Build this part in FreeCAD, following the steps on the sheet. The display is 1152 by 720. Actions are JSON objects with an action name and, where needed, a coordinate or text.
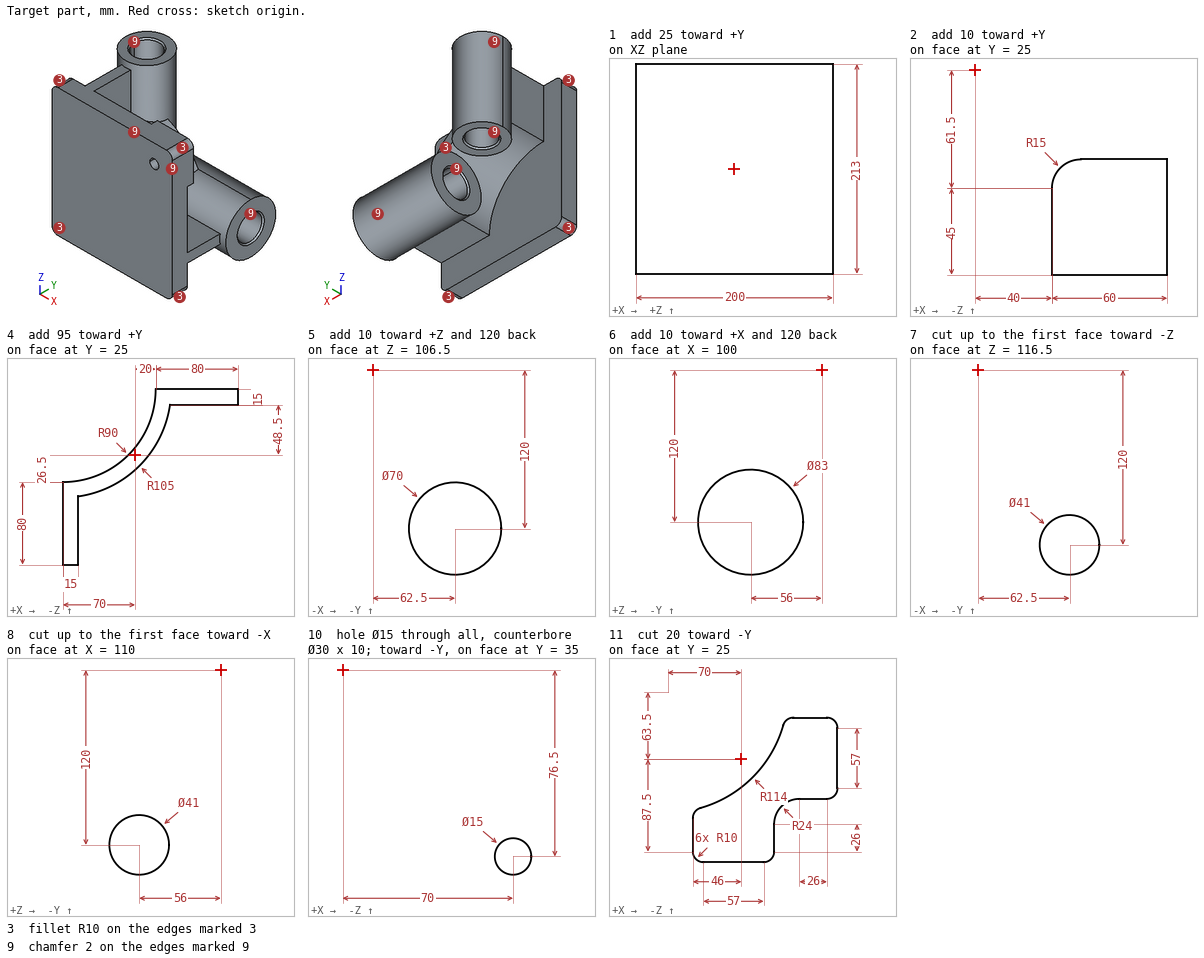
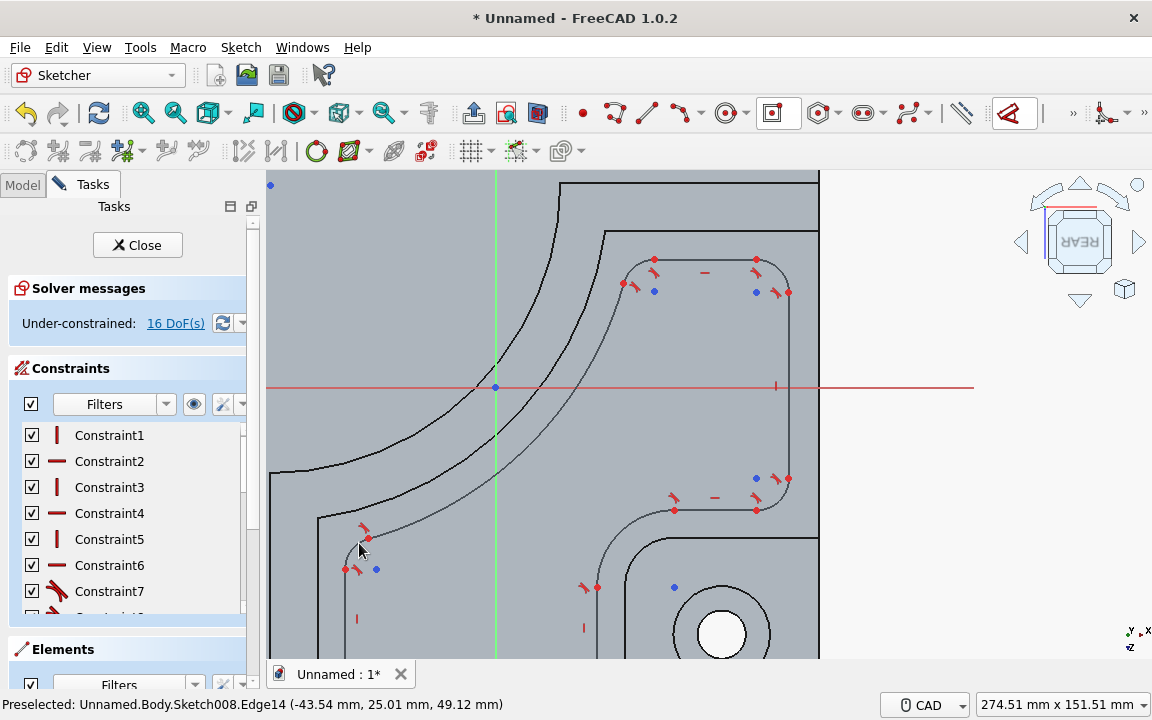
{"action": "scroll", "coordinate": [787, 279], "scroll_direction": "down", "scroll_amount": 2}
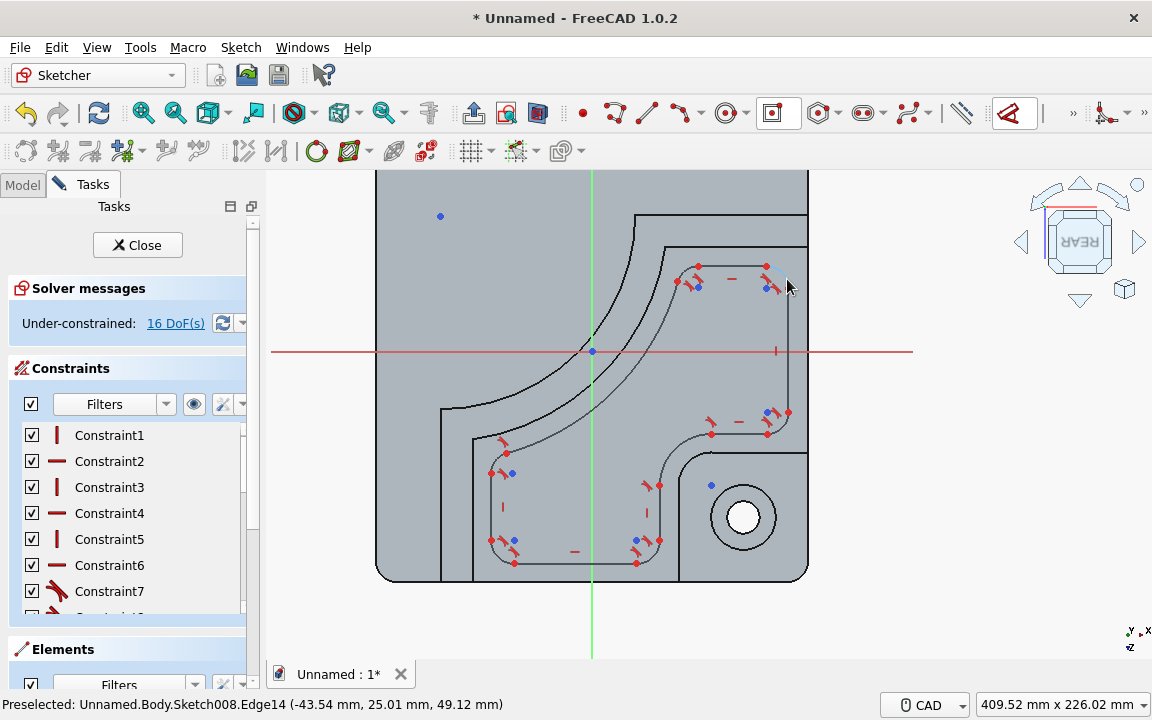
{"action": "scroll", "coordinate": [494, 551], "scroll_direction": "up", "scroll_amount": 2}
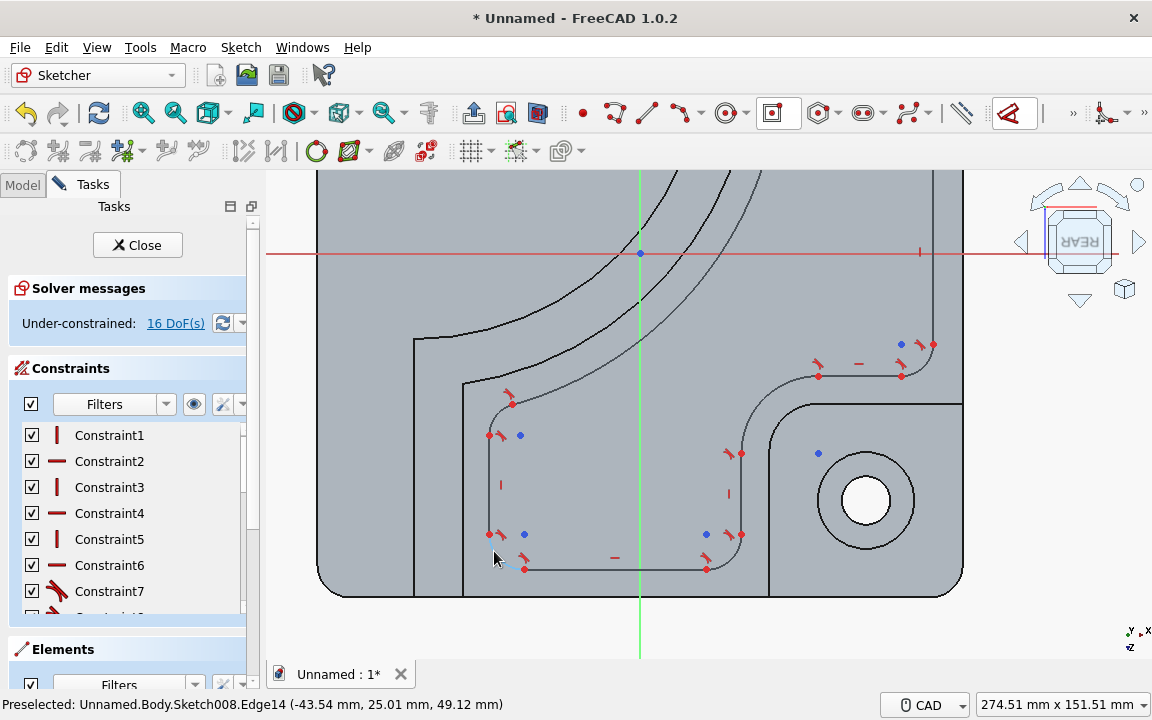
{"action": "left_click", "coordinate": [493, 551]}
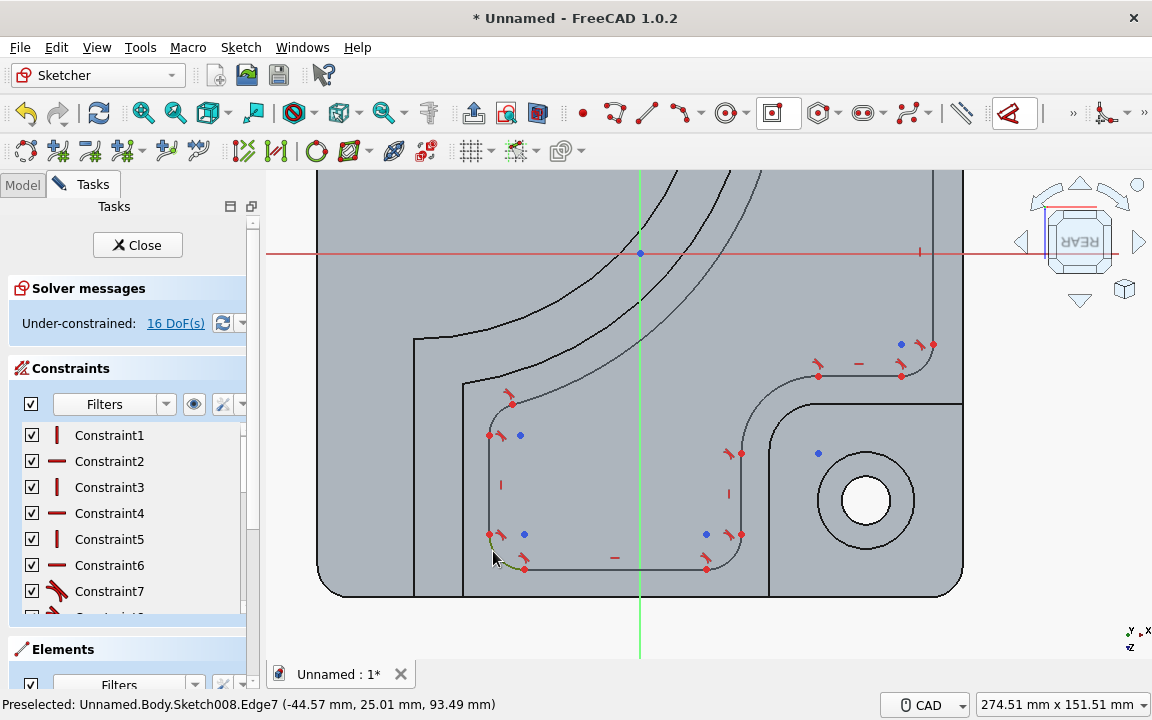
{"action": "left_click", "coordinate": [722, 566]}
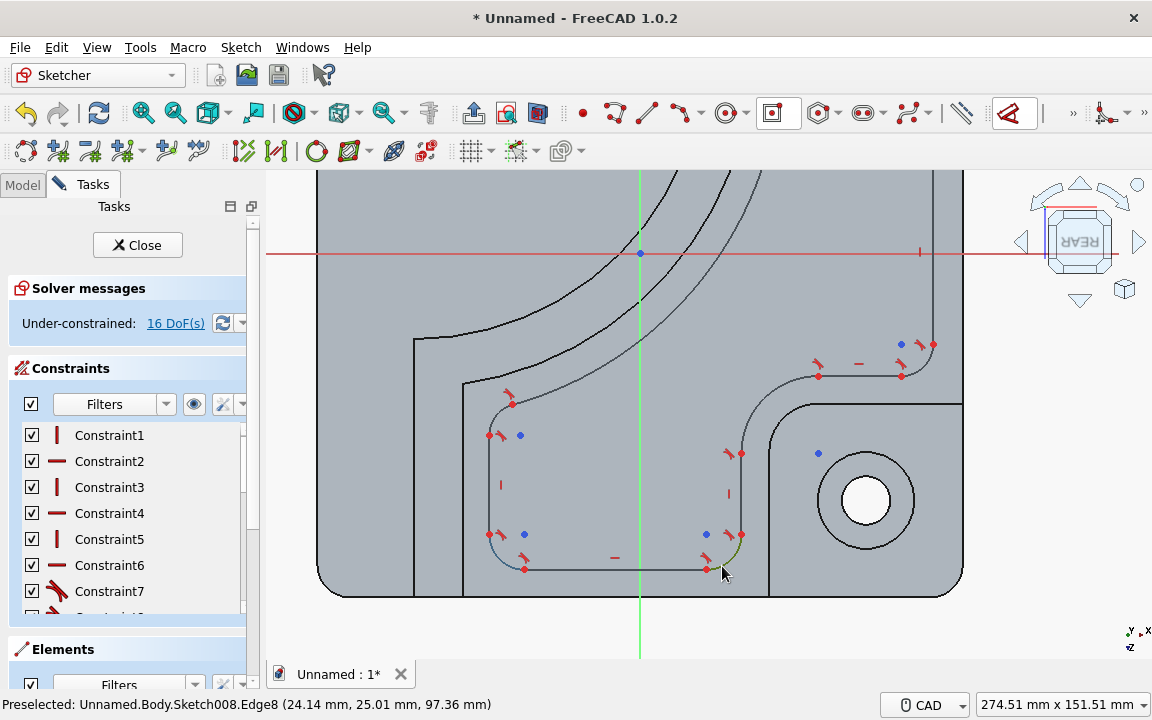
{"action": "left_click", "coordinate": [916, 373]}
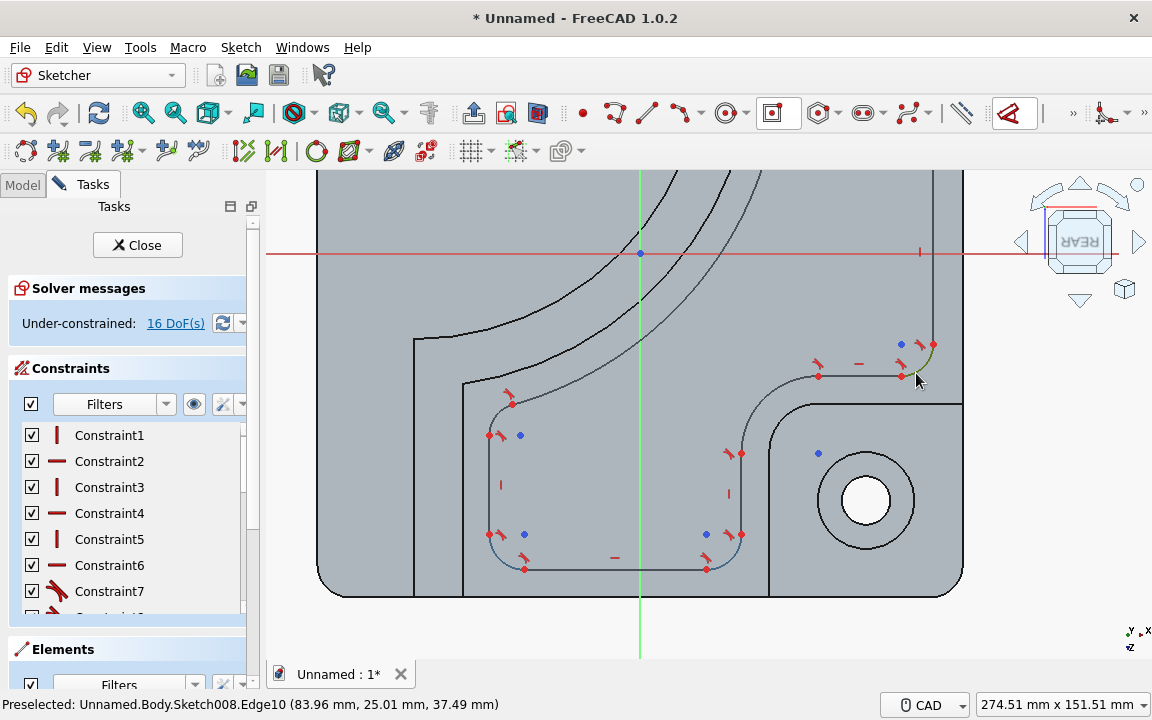
{"action": "scroll", "coordinate": [494, 551], "scroll_direction": "down", "scroll_amount": 2}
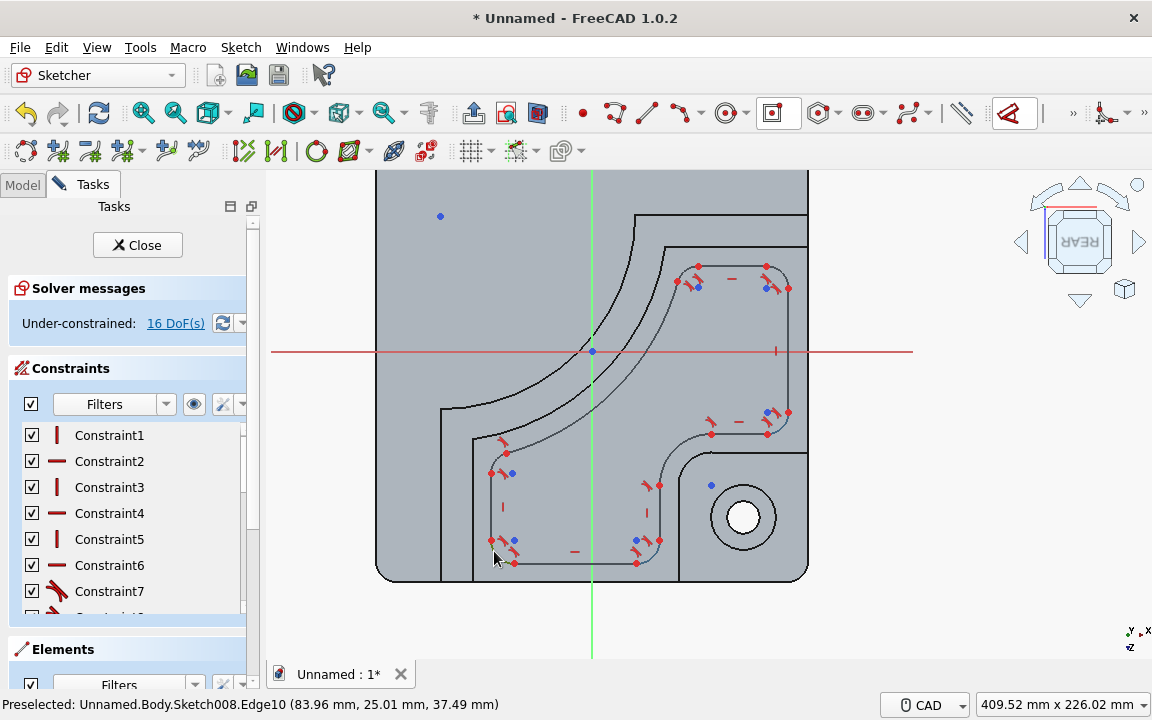
{"action": "scroll", "coordinate": [786, 278], "scroll_direction": "up", "scroll_amount": 2}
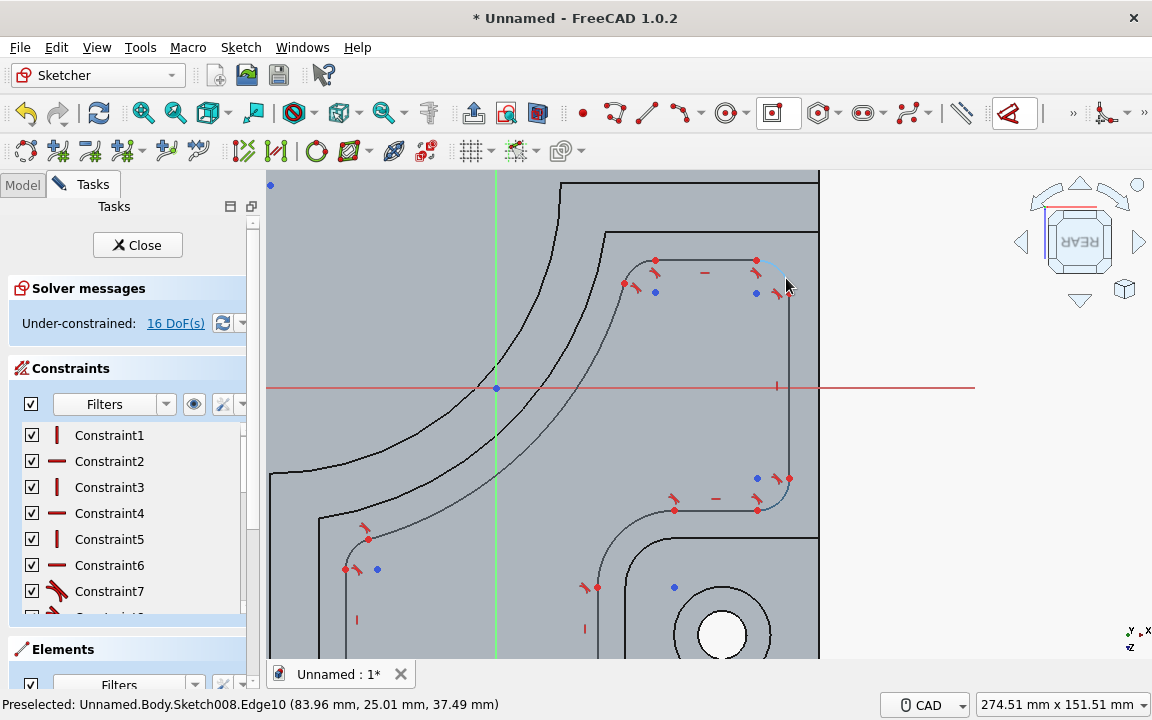
{"action": "left_click", "coordinate": [786, 278]}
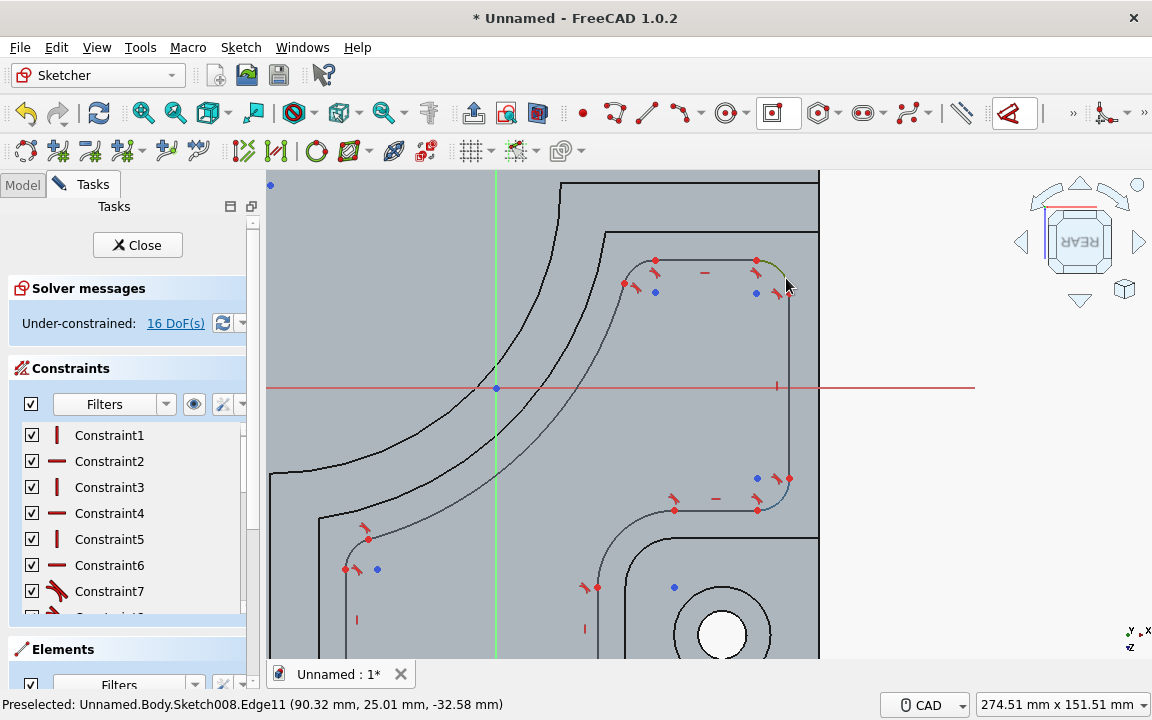
{"action": "left_click", "coordinate": [643, 263]}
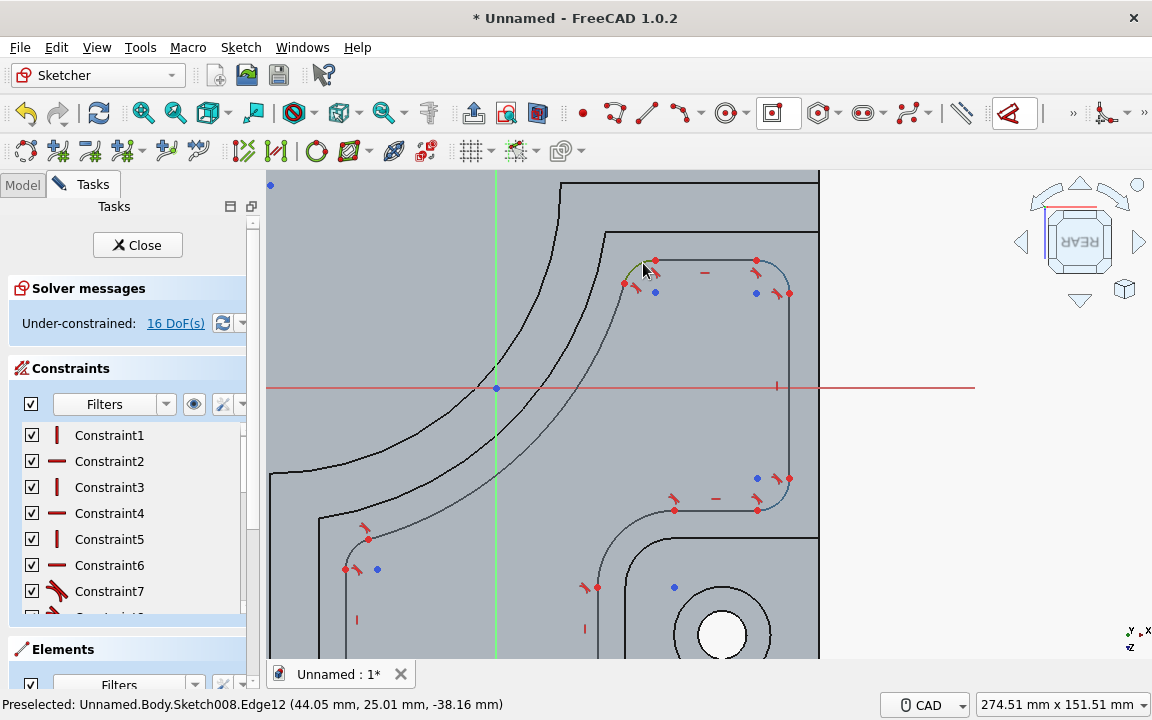
{"action": "left_click", "coordinate": [358, 545]}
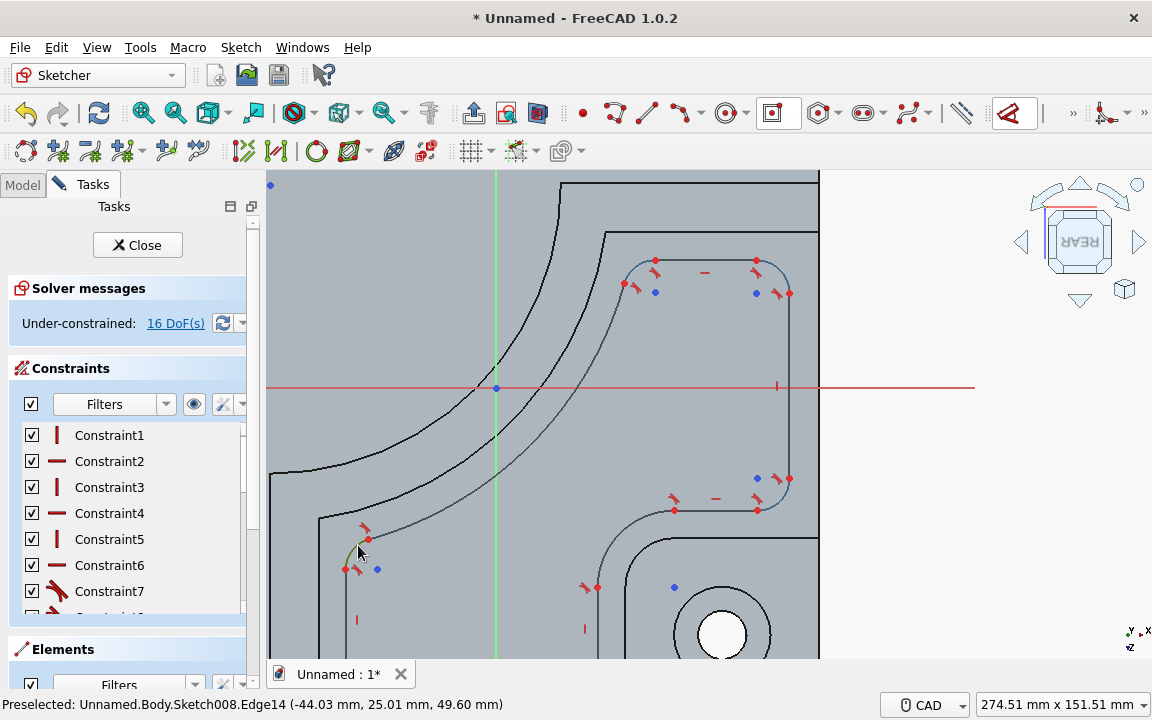
{"action": "key", "text": "e"}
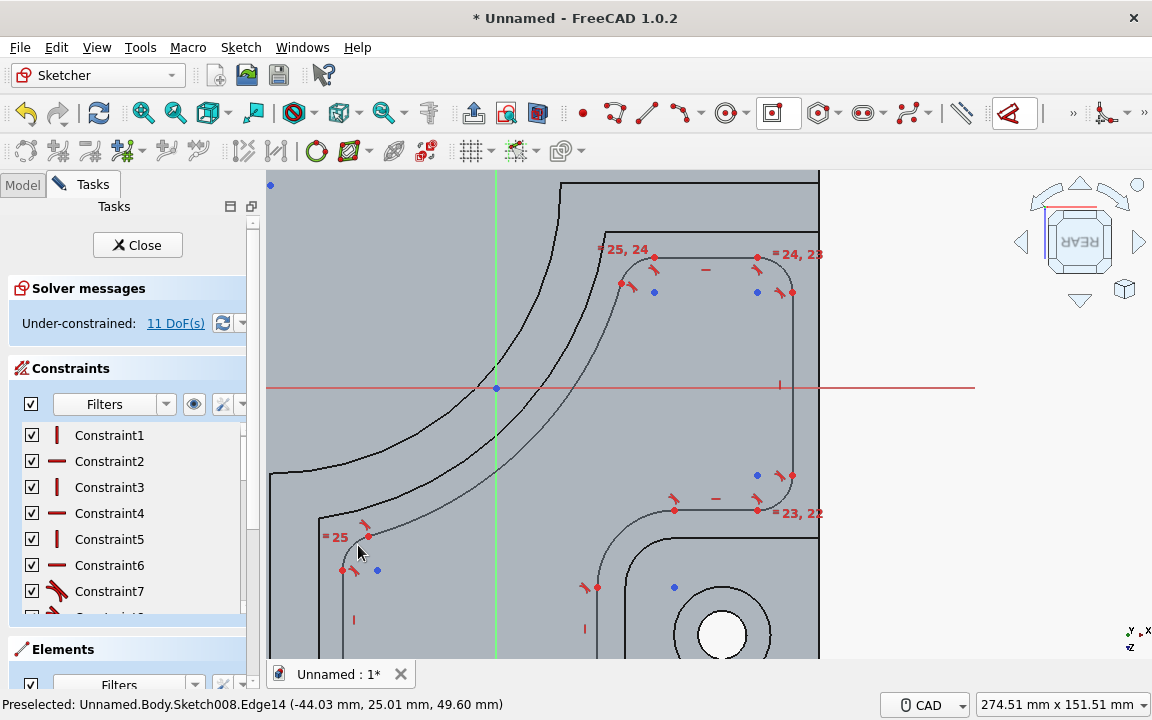
{"action": "scroll", "coordinate": [786, 278], "scroll_direction": "down", "scroll_amount": 2}